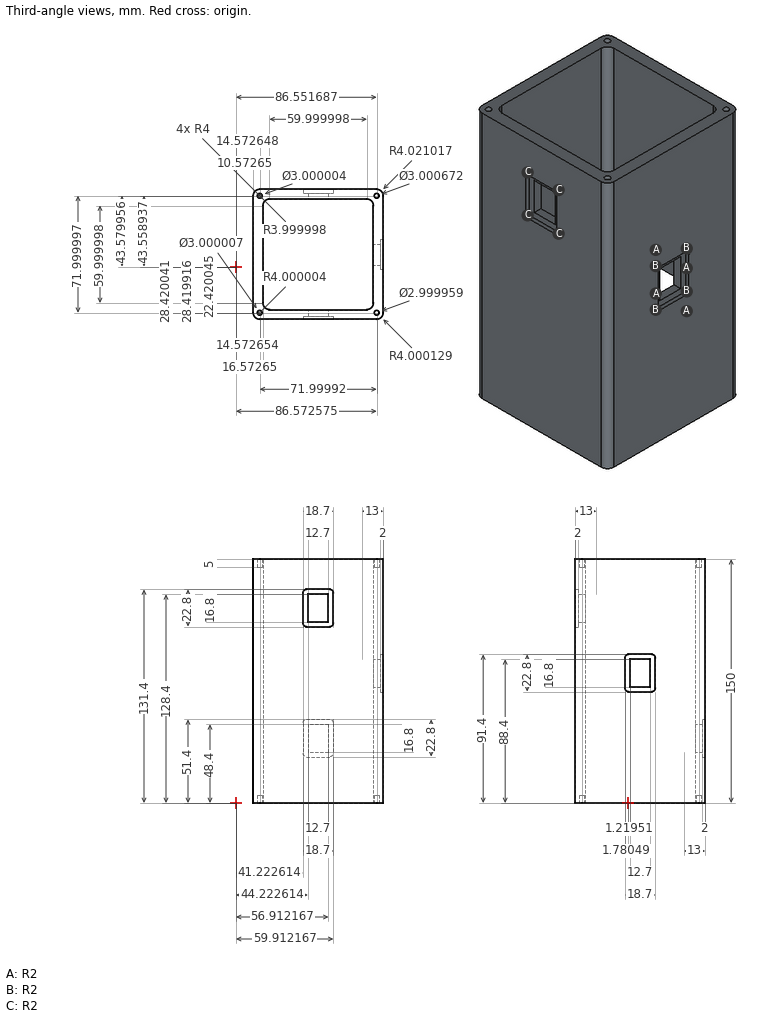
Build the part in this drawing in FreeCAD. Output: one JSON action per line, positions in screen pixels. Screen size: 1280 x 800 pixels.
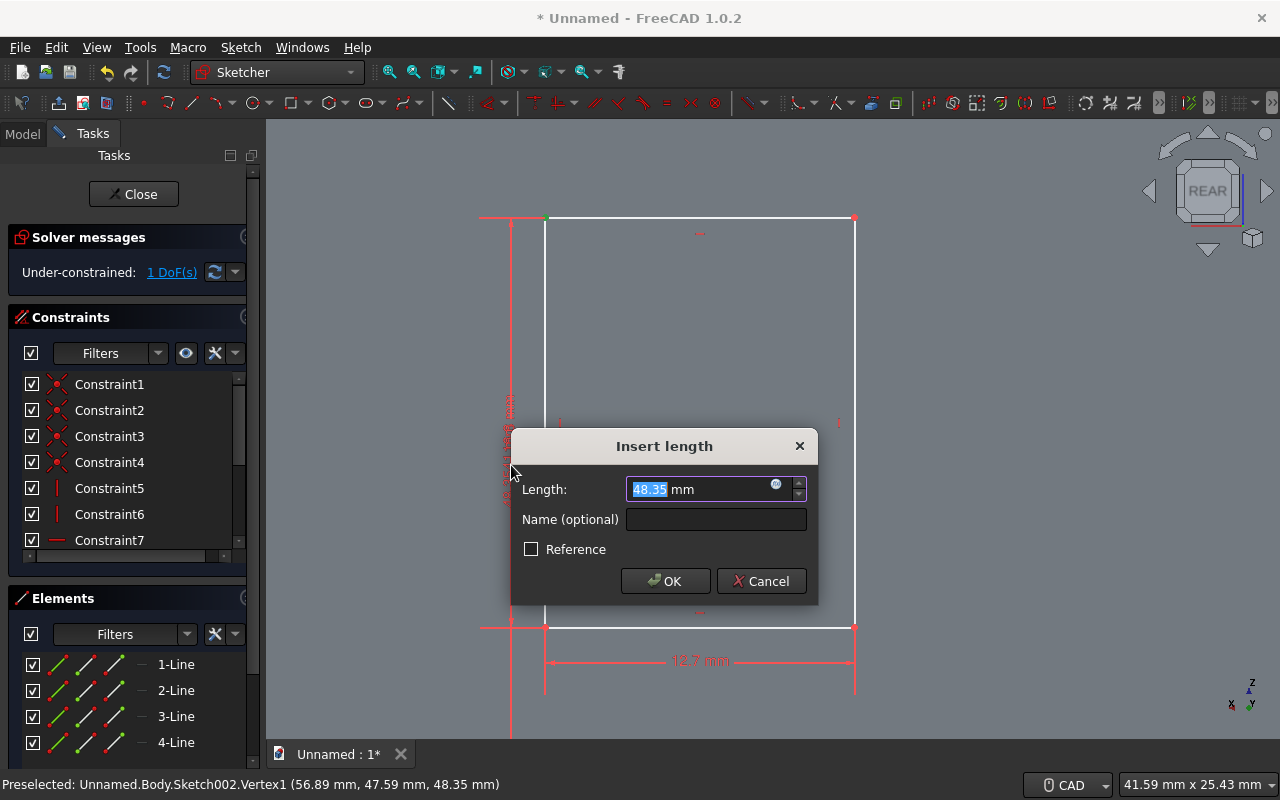
{"action": "type", "text": "48.4"}
{"action": "key", "text": "Return"}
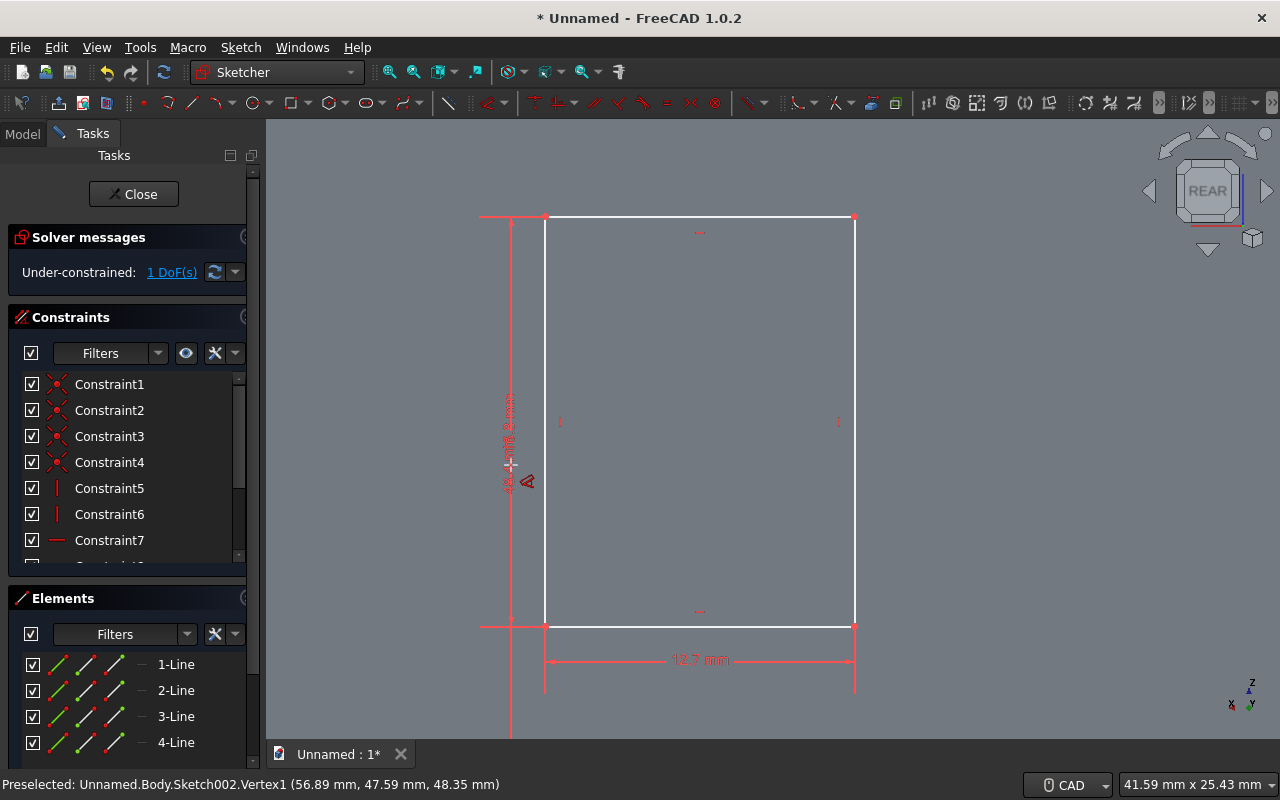
{"action": "left_click", "coordinate": [545, 217]}
{"action": "left_click", "coordinate": [830, 183]}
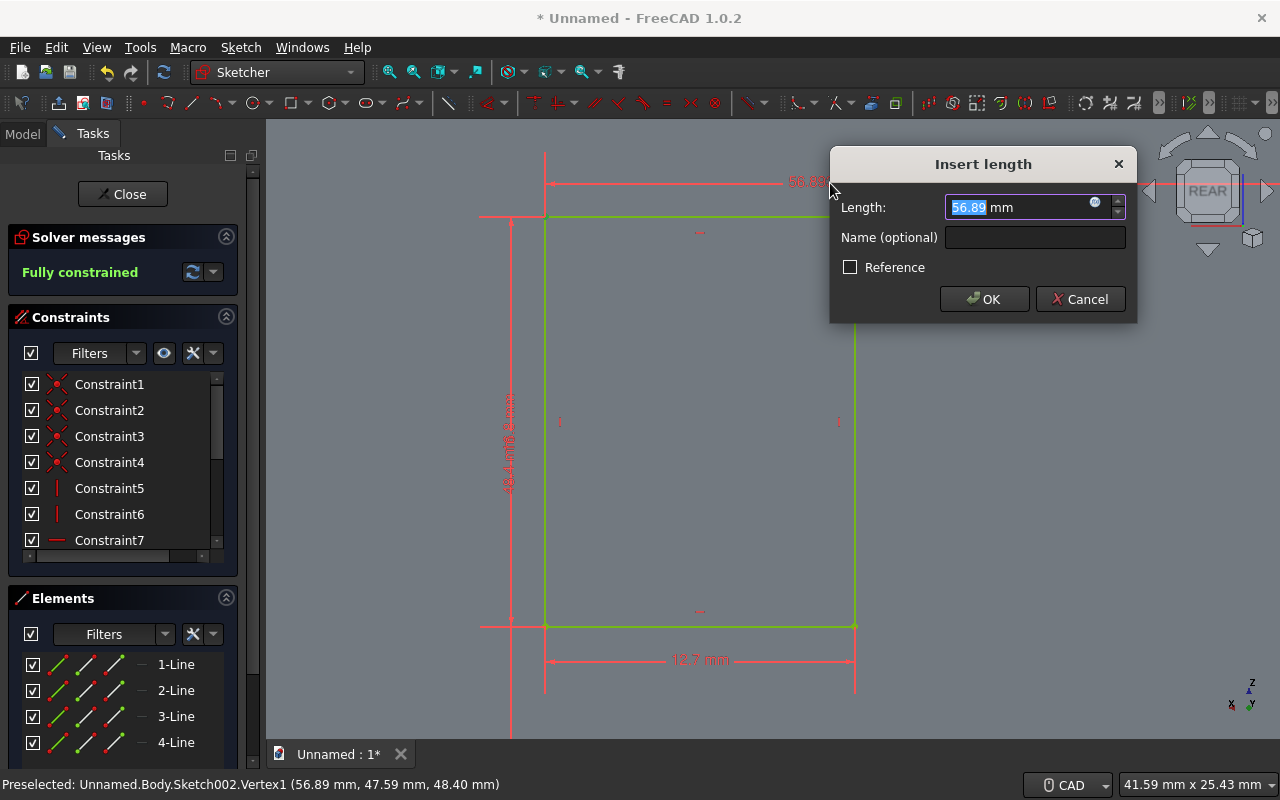
{"action": "type", "text": "56.912167"}
{"action": "key", "text": "Return"}
{"action": "key", "text": "Escape"}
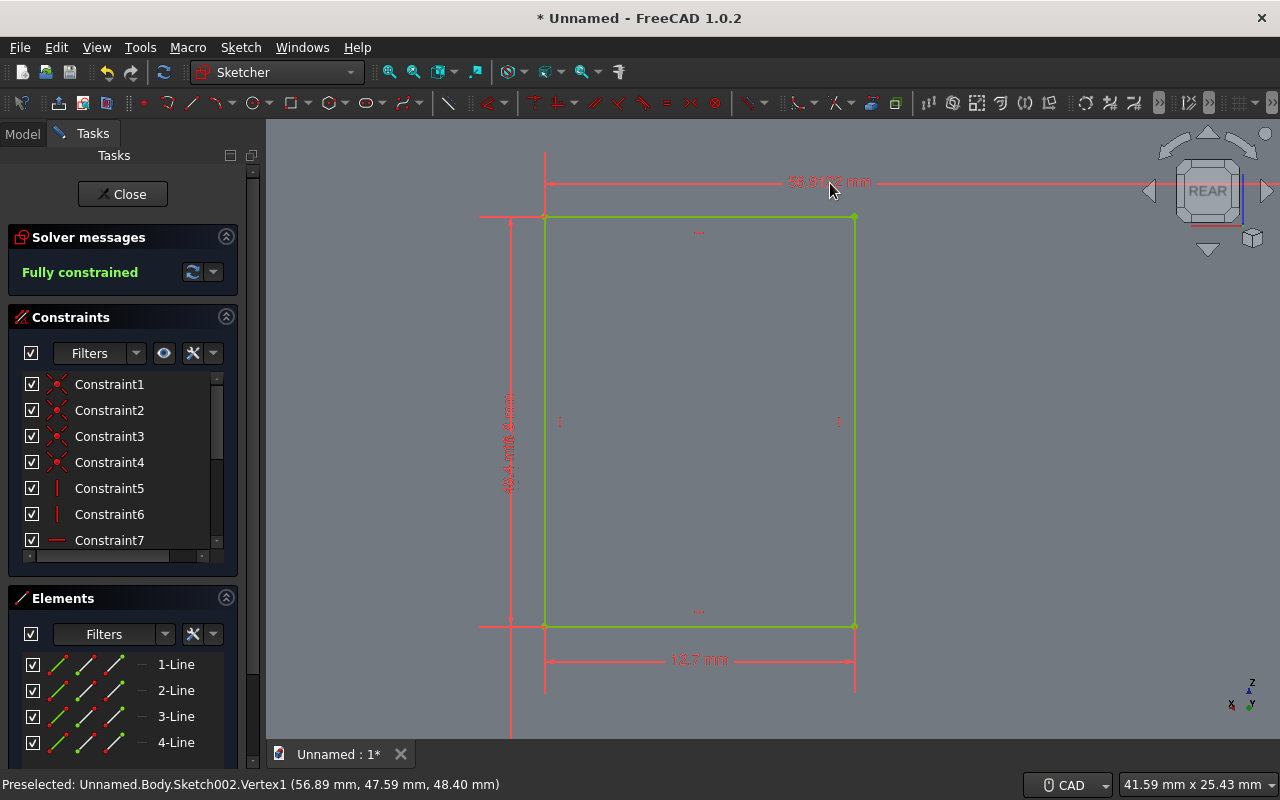
{"action": "left_click", "coordinate": [123, 194]}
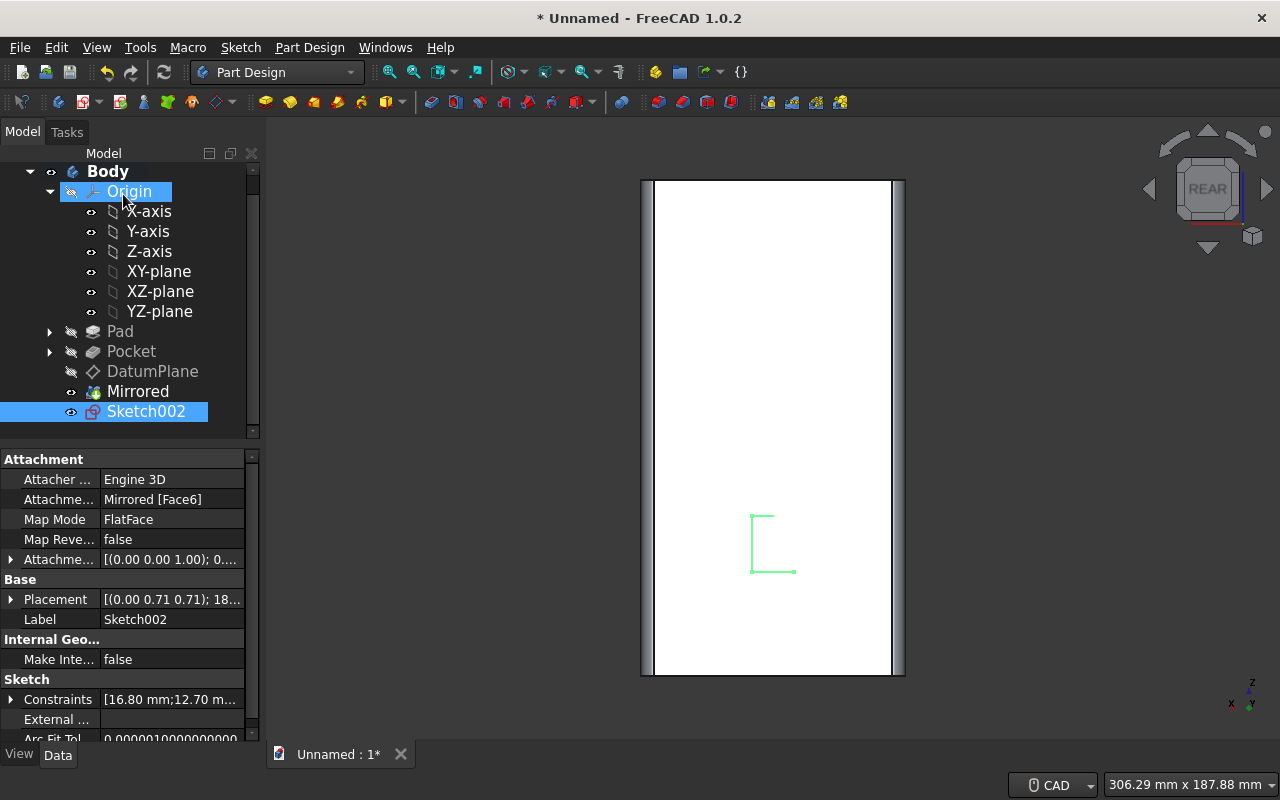
{"action": "left_click", "coordinate": [432, 102]}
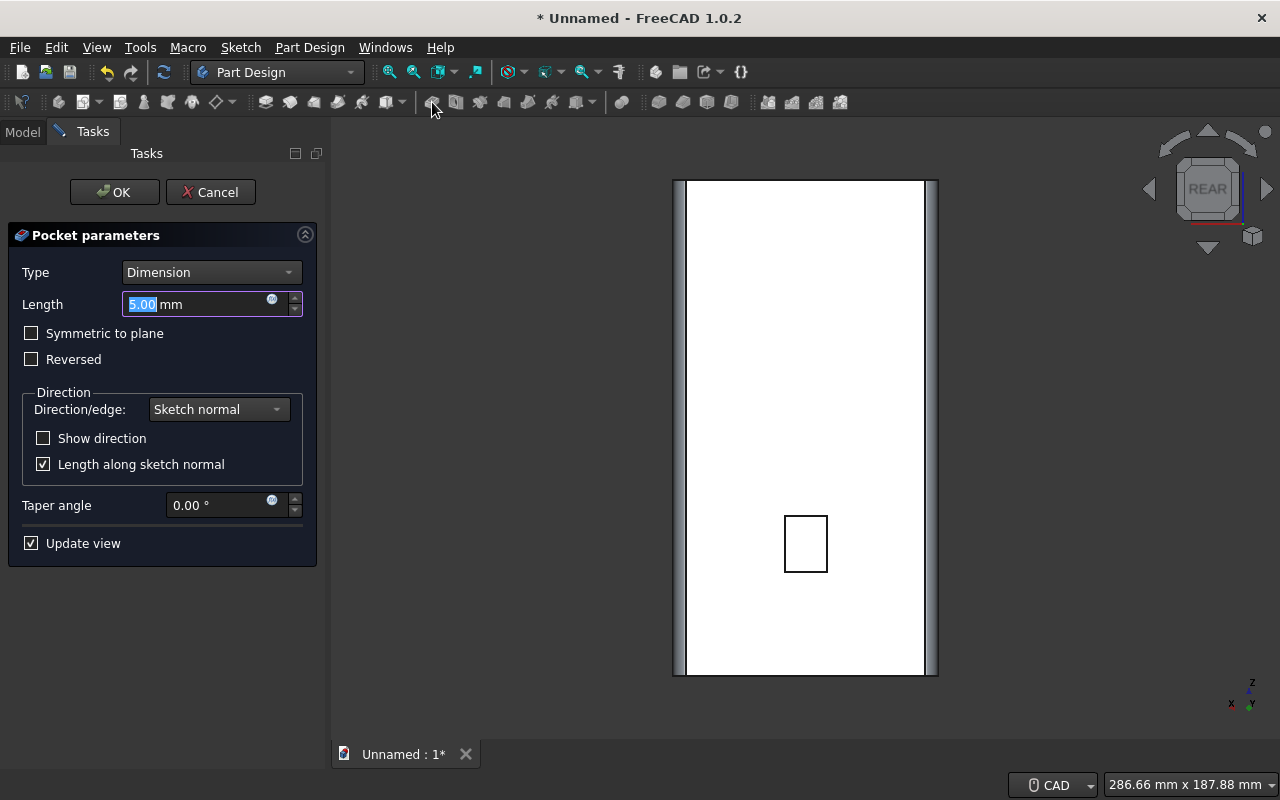
{"action": "type", "text": "13"}
{"action": "key", "text": "Tab"}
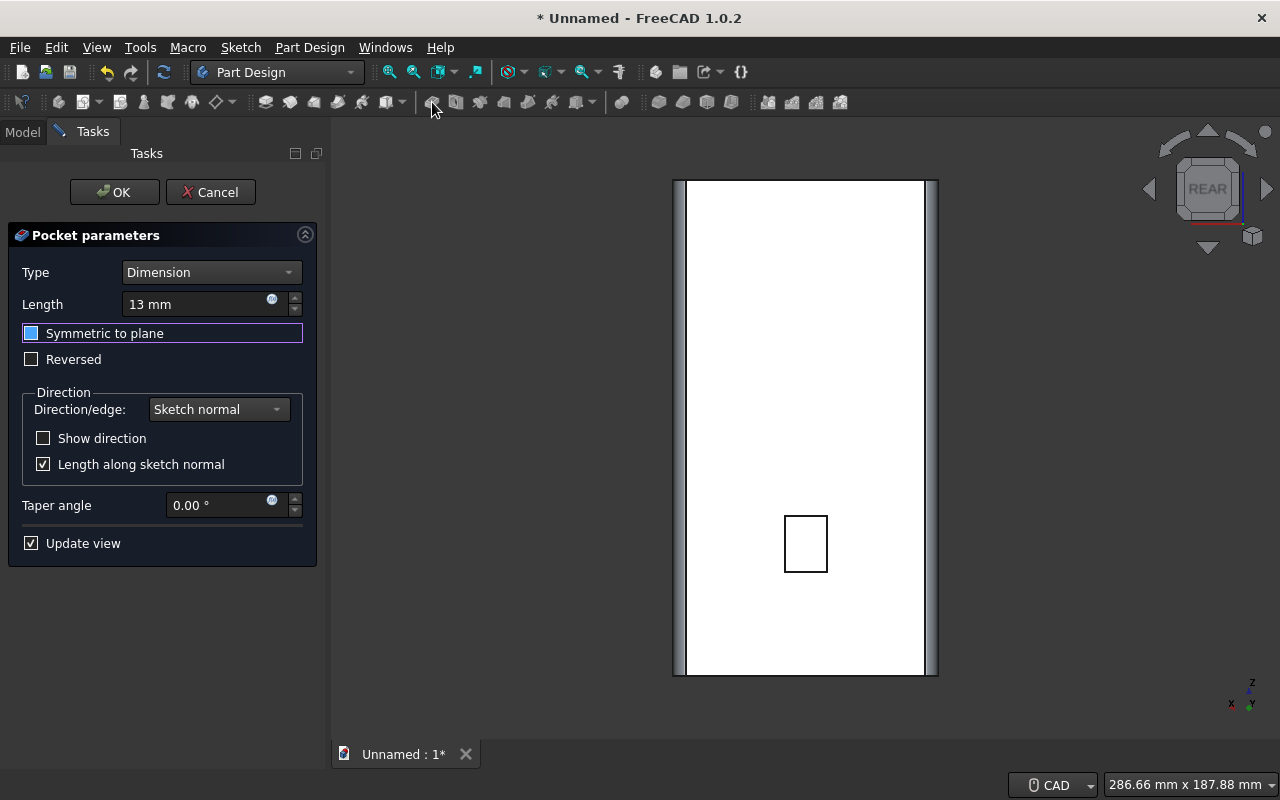
{"action": "left_click", "coordinate": [115, 192]}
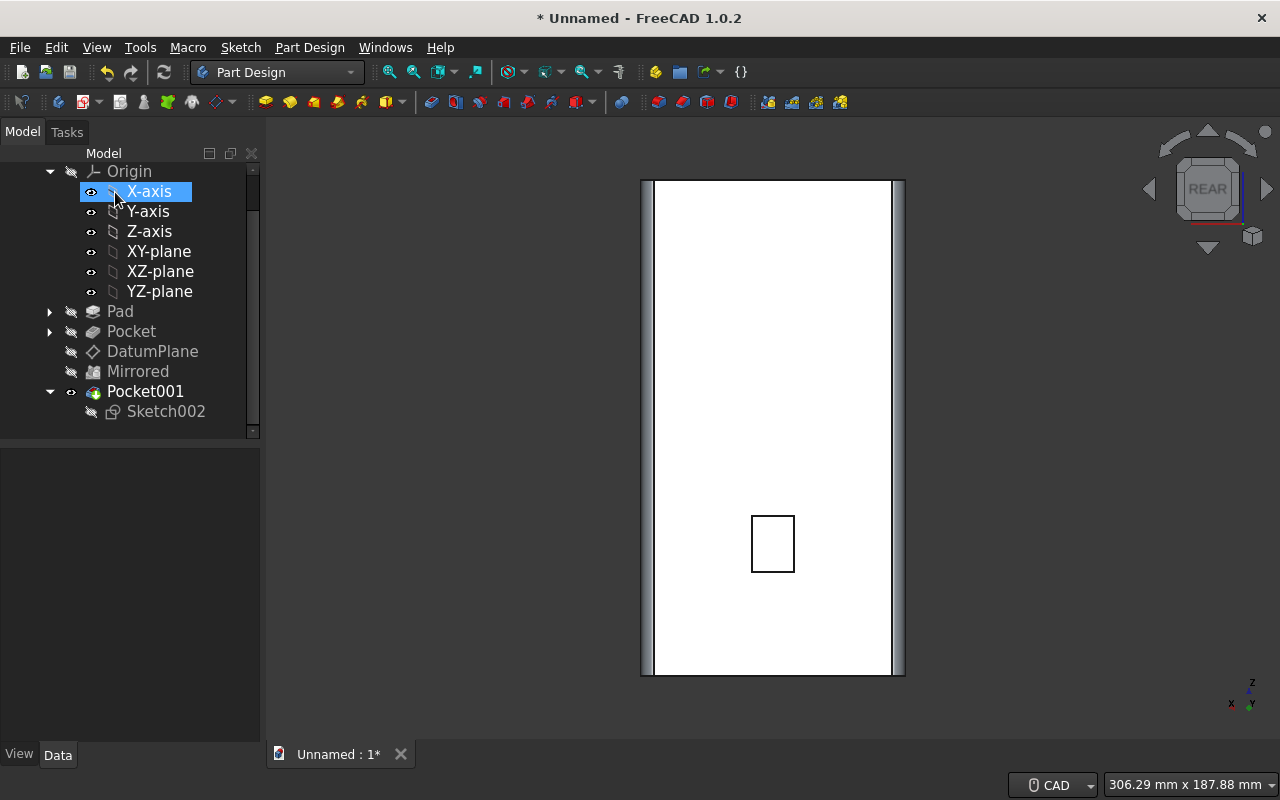
{"action": "key", "text": "0"}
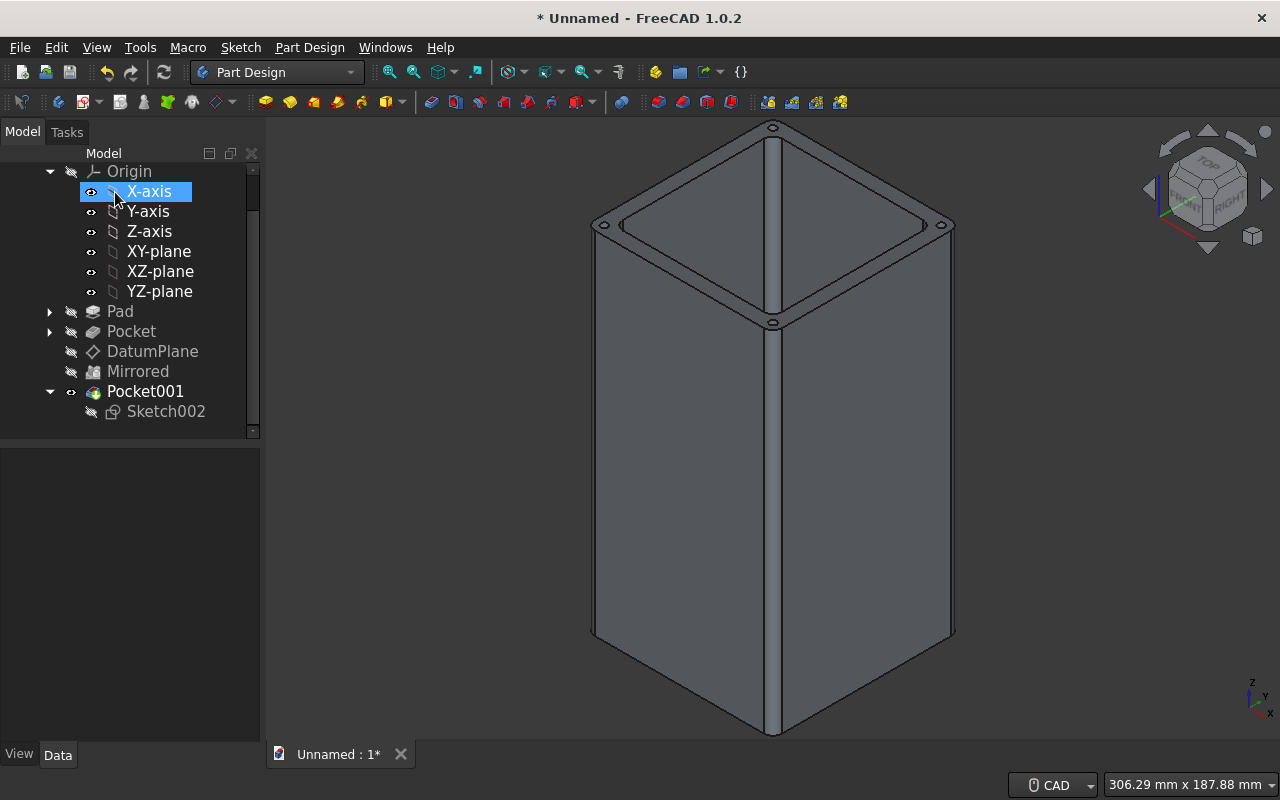
{"action": "left_click", "coordinate": [390, 72]}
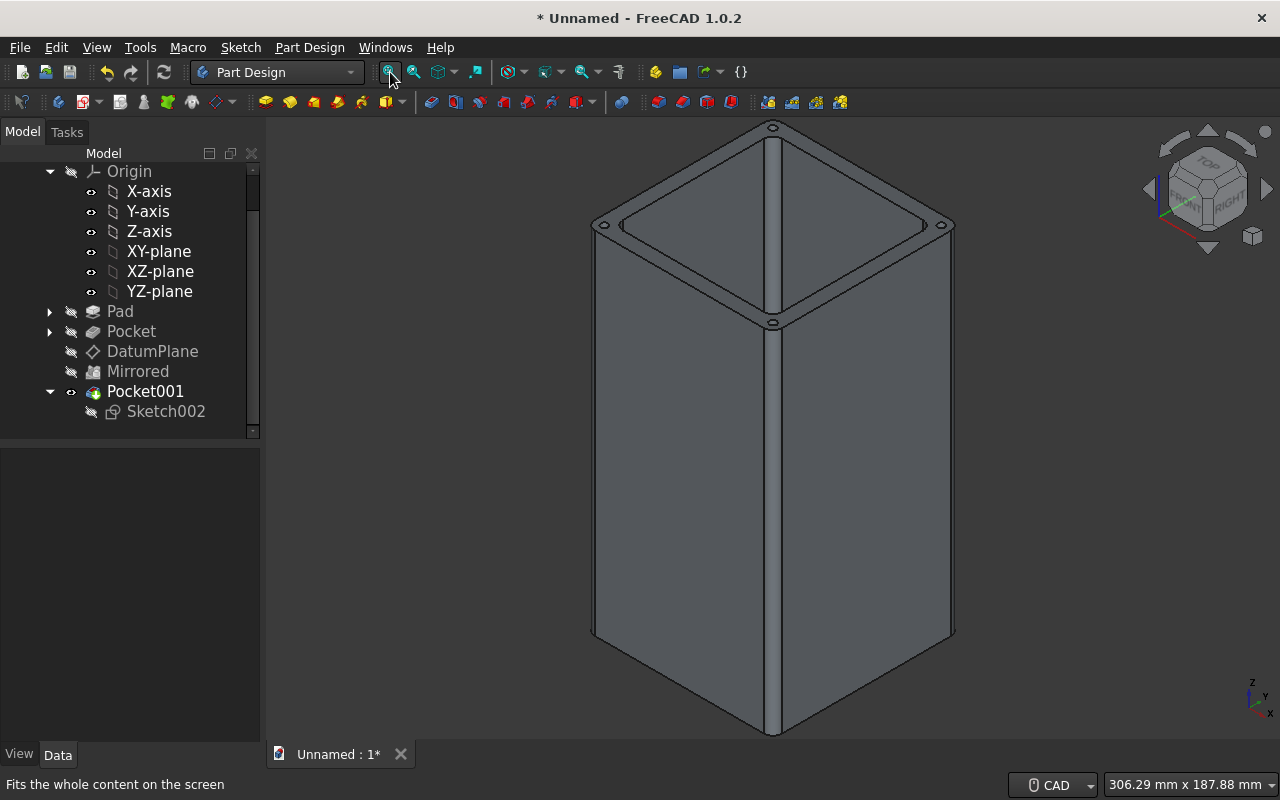
{"action": "left_click", "coordinate": [867, 423]}